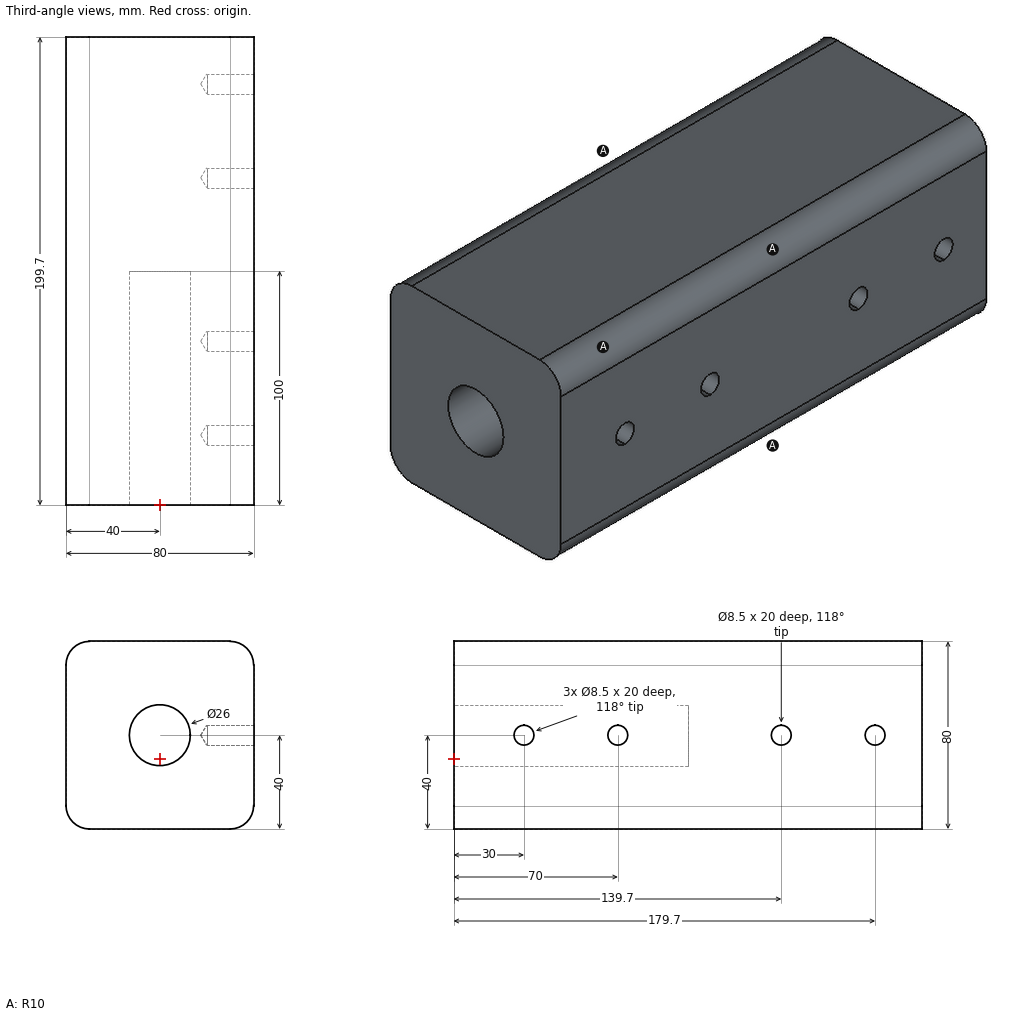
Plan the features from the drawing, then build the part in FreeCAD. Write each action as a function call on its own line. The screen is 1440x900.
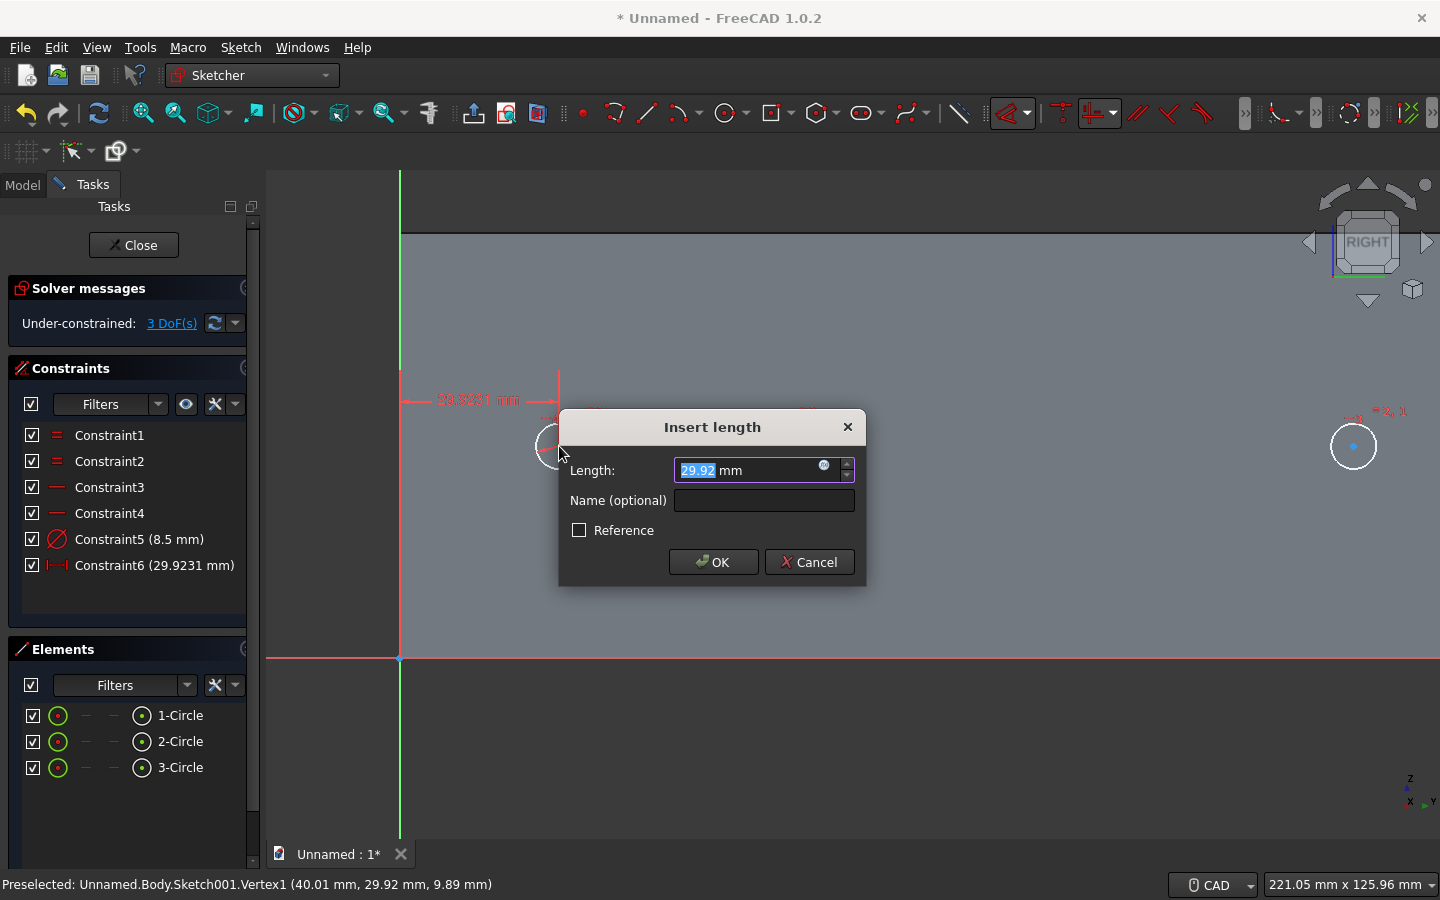
text(30)
key(Return)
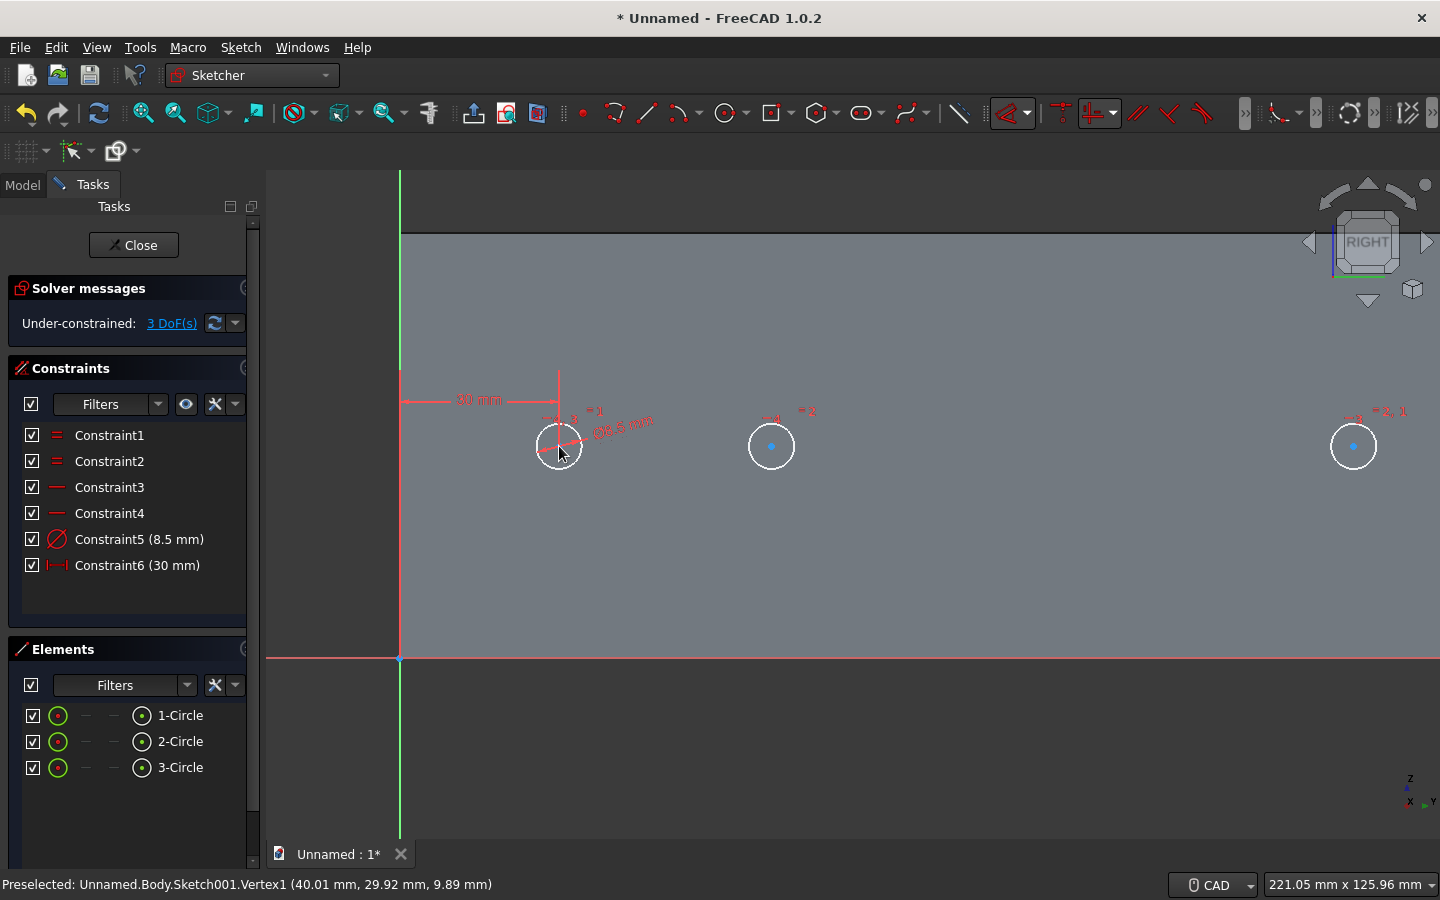
click(559, 446)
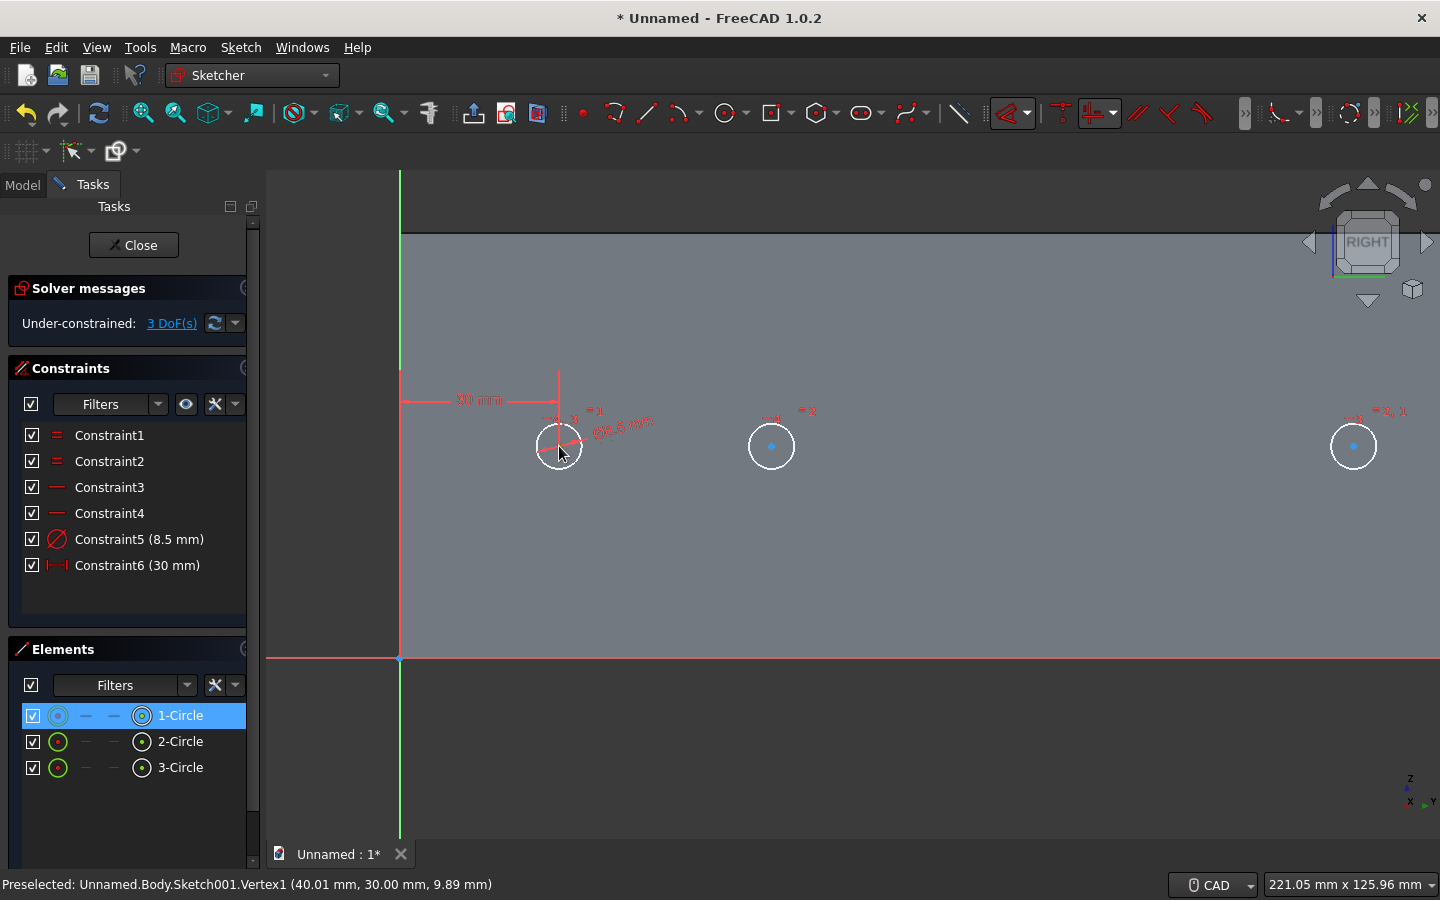
key(i)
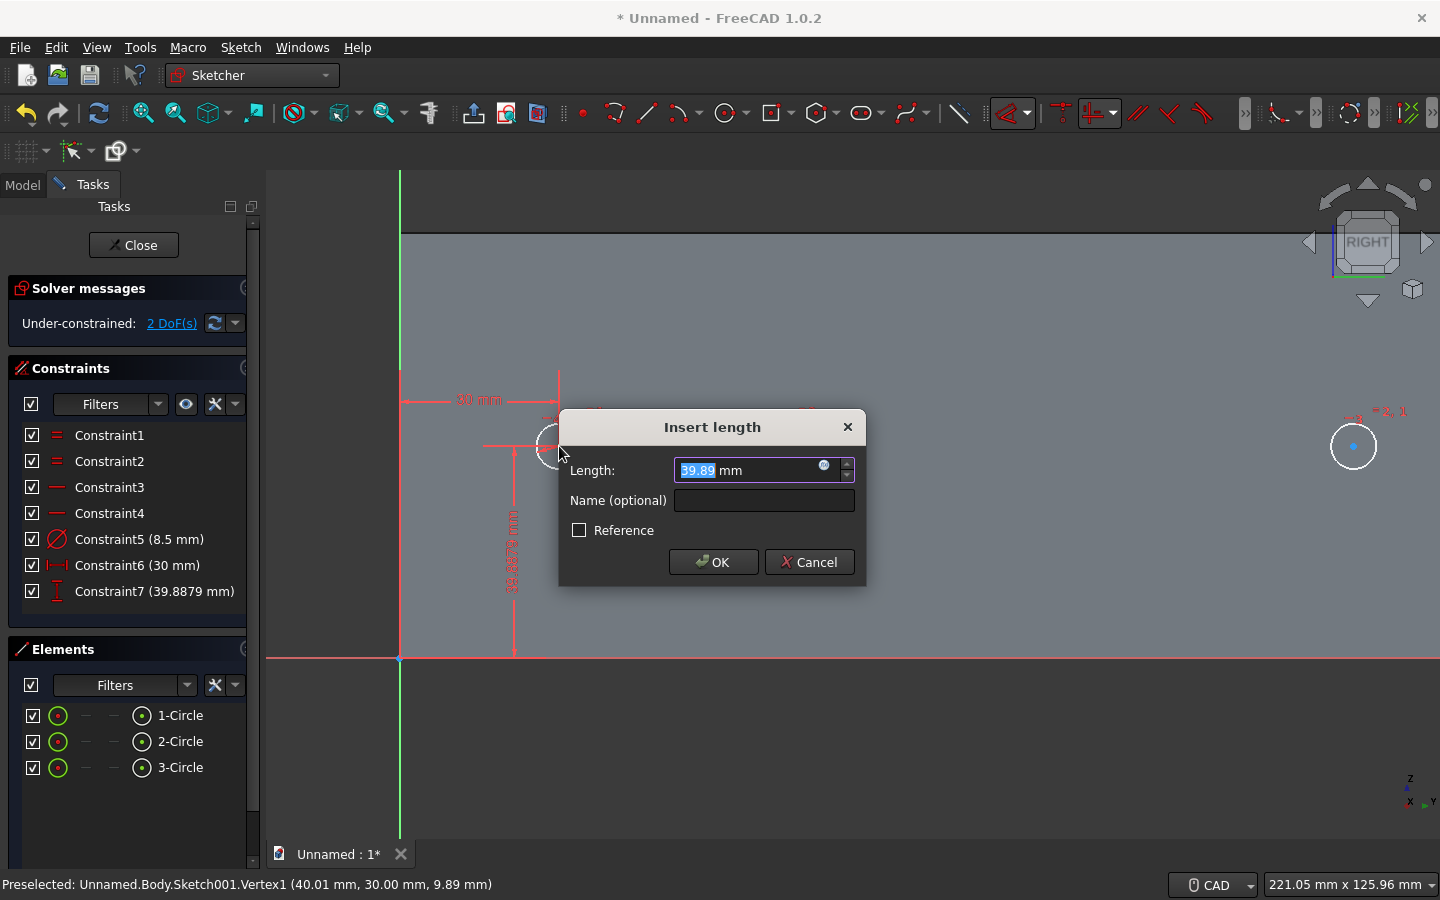
text(40)
key(Return)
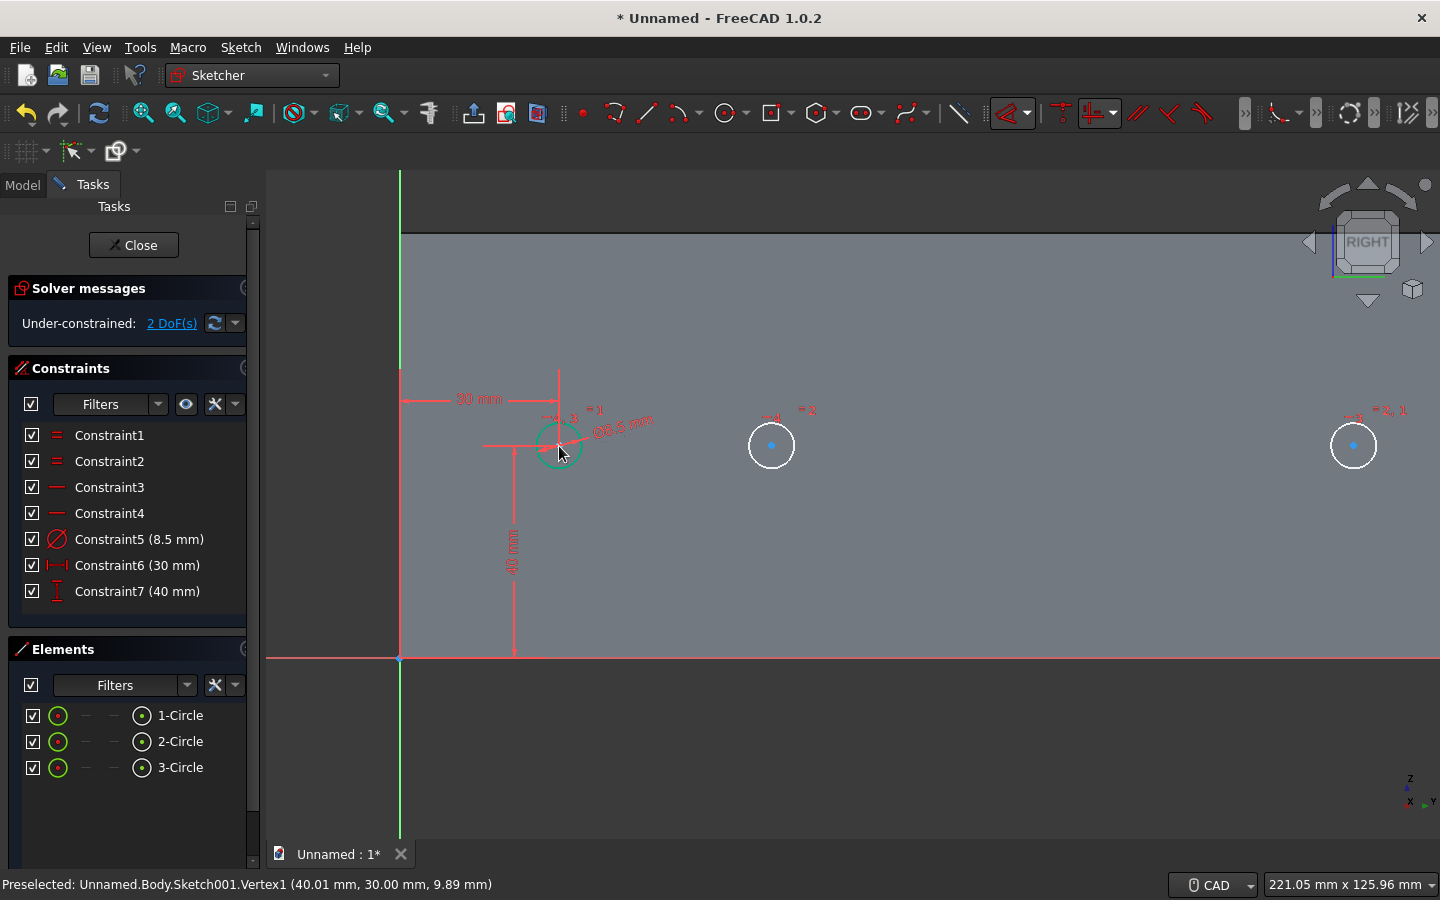
click(772, 446)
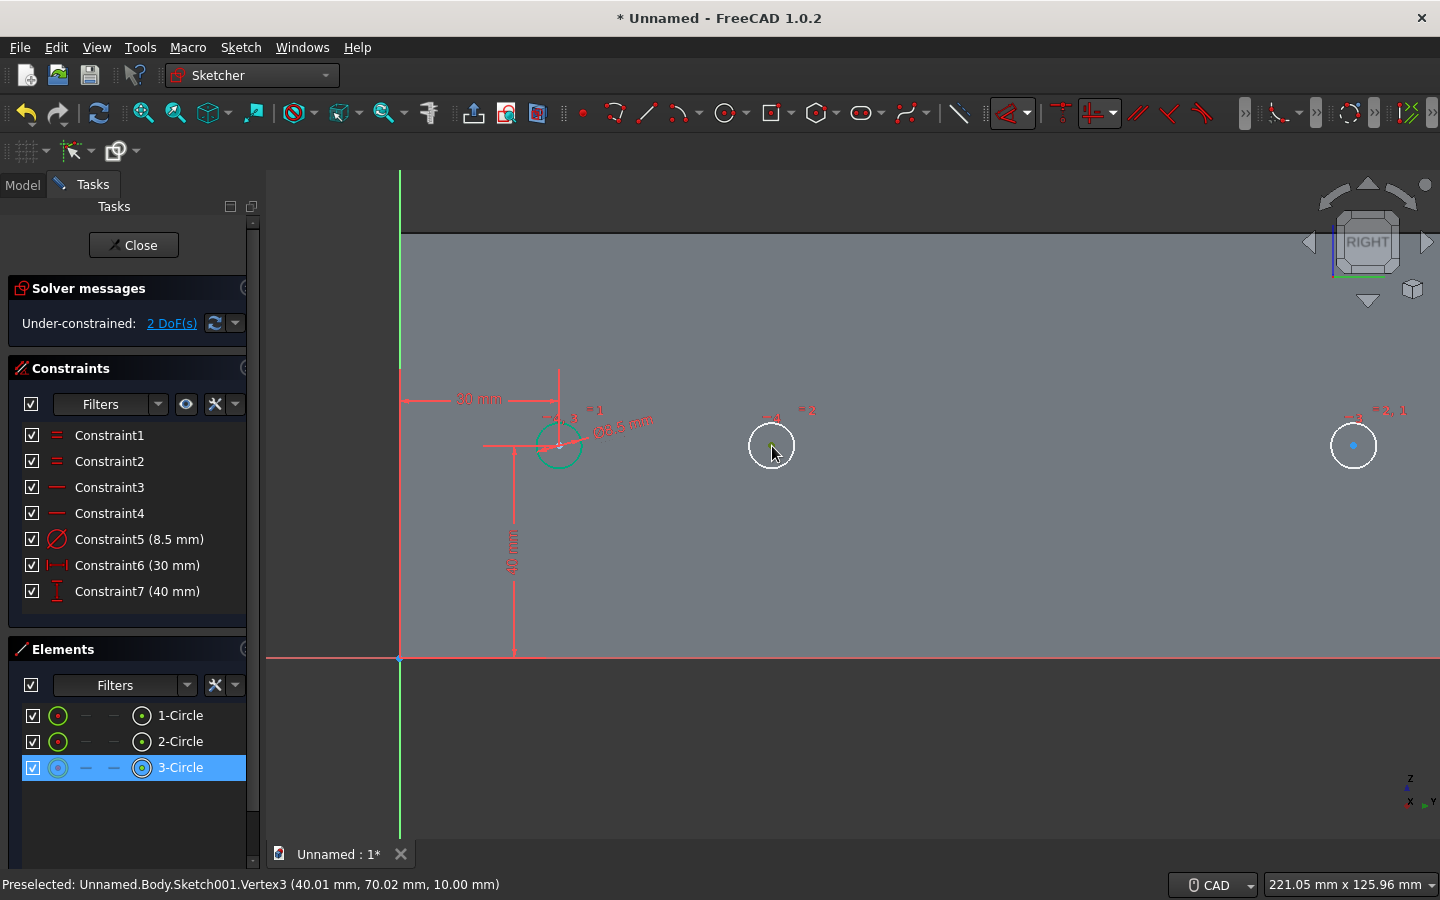
key(l)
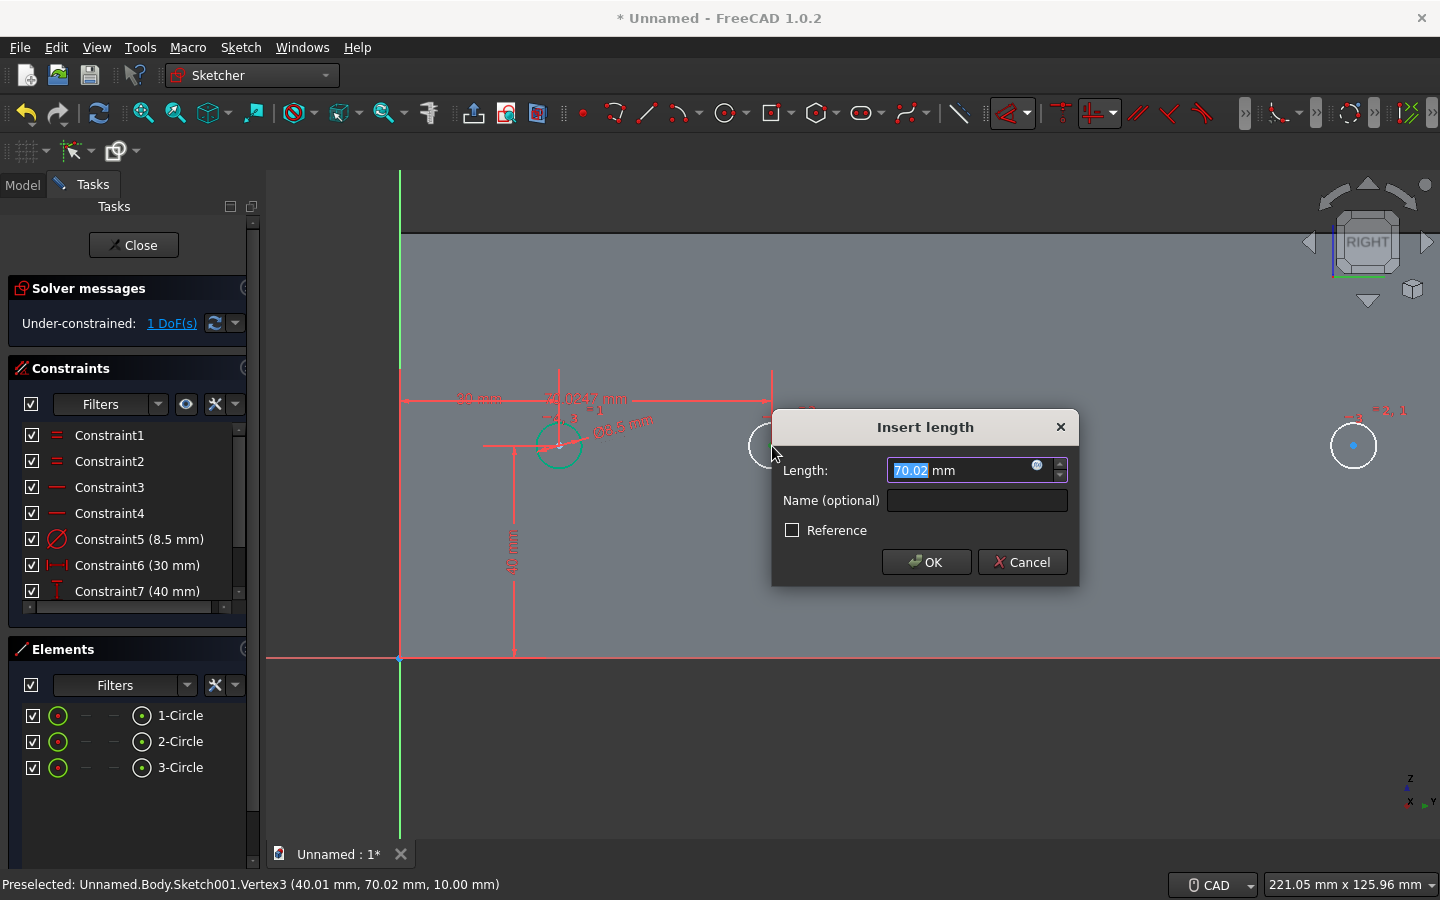
text(70)
key(Return)